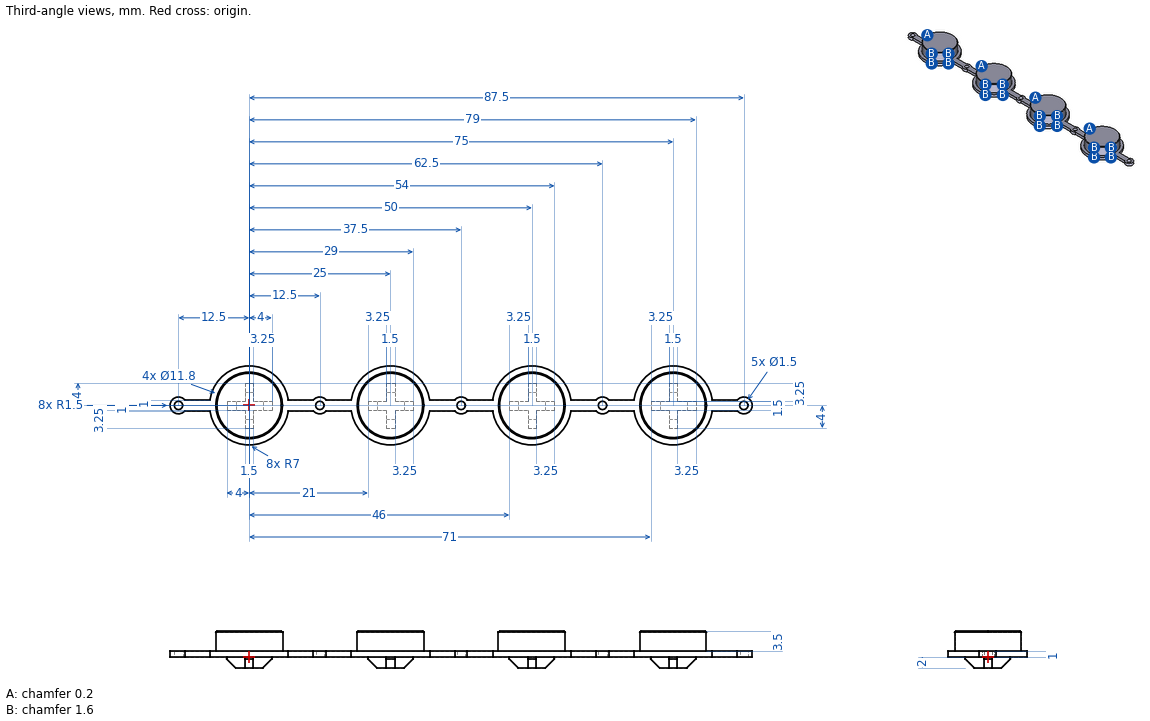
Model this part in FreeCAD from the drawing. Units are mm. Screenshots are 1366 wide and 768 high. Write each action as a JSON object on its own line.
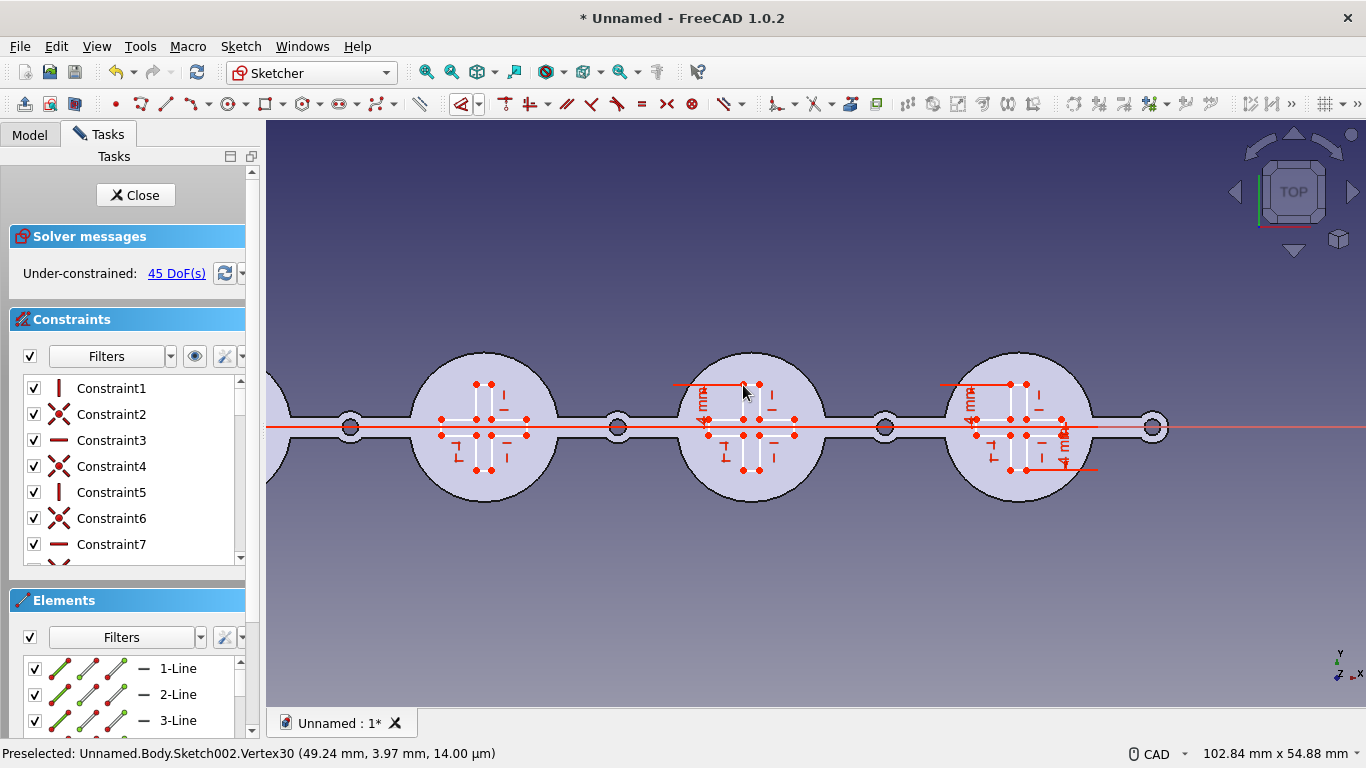
{"action": "left_click", "coordinate": [760, 471]}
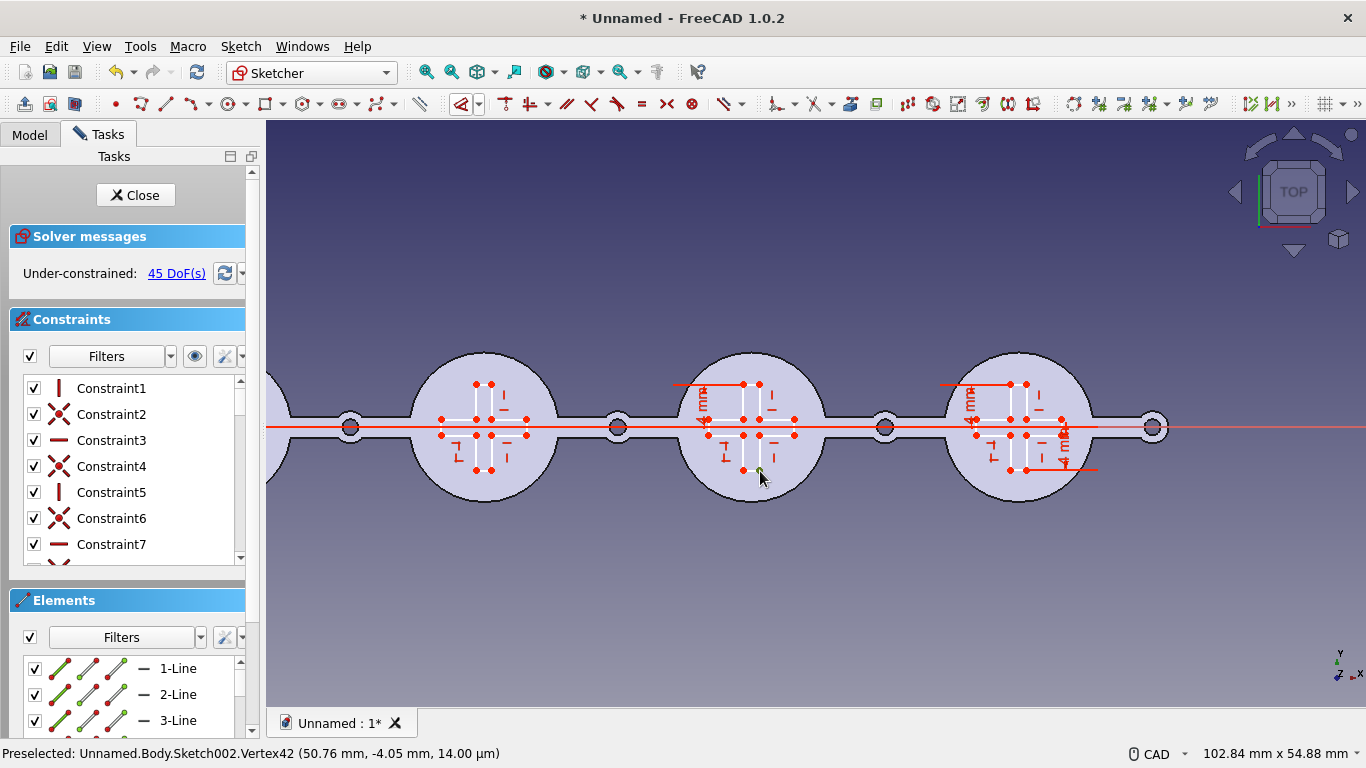
{"action": "left_click", "coordinate": [478, 104]}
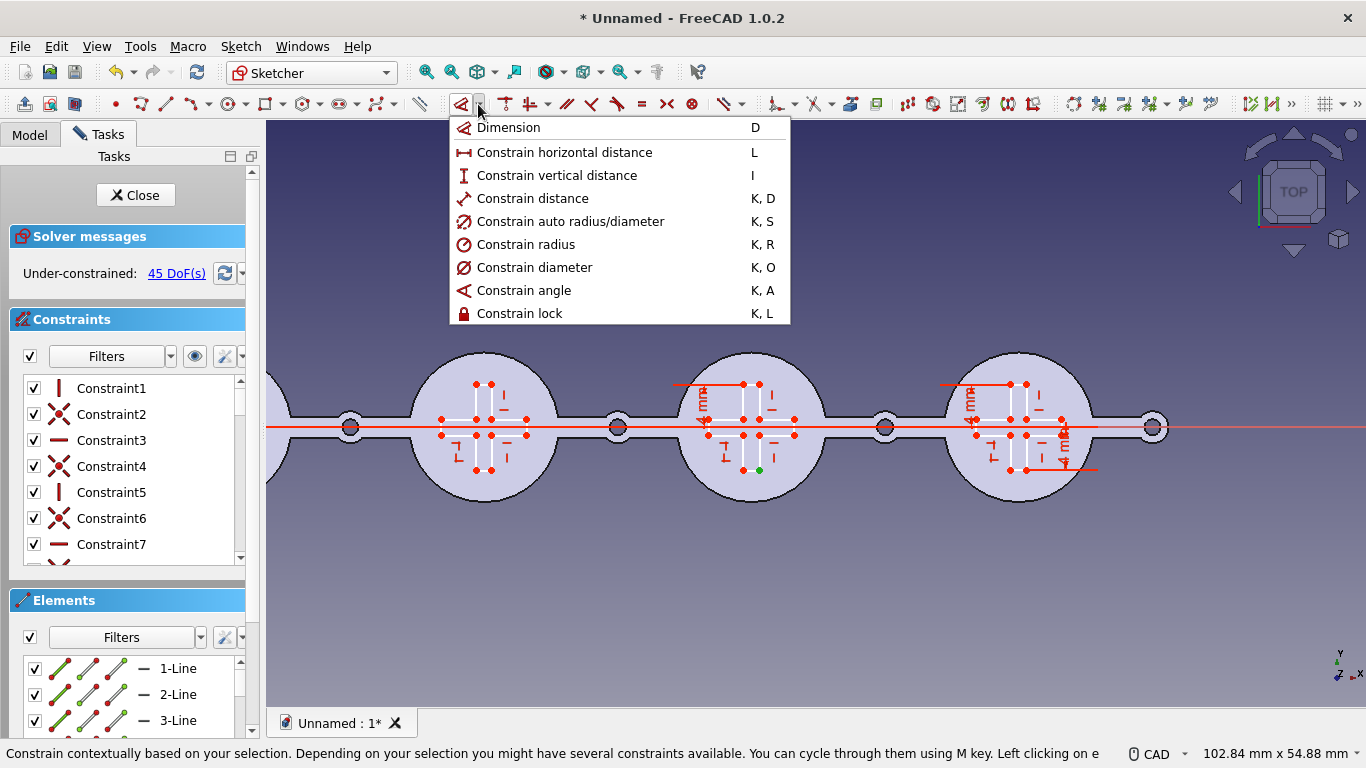
{"action": "left_click", "coordinate": [620, 176]}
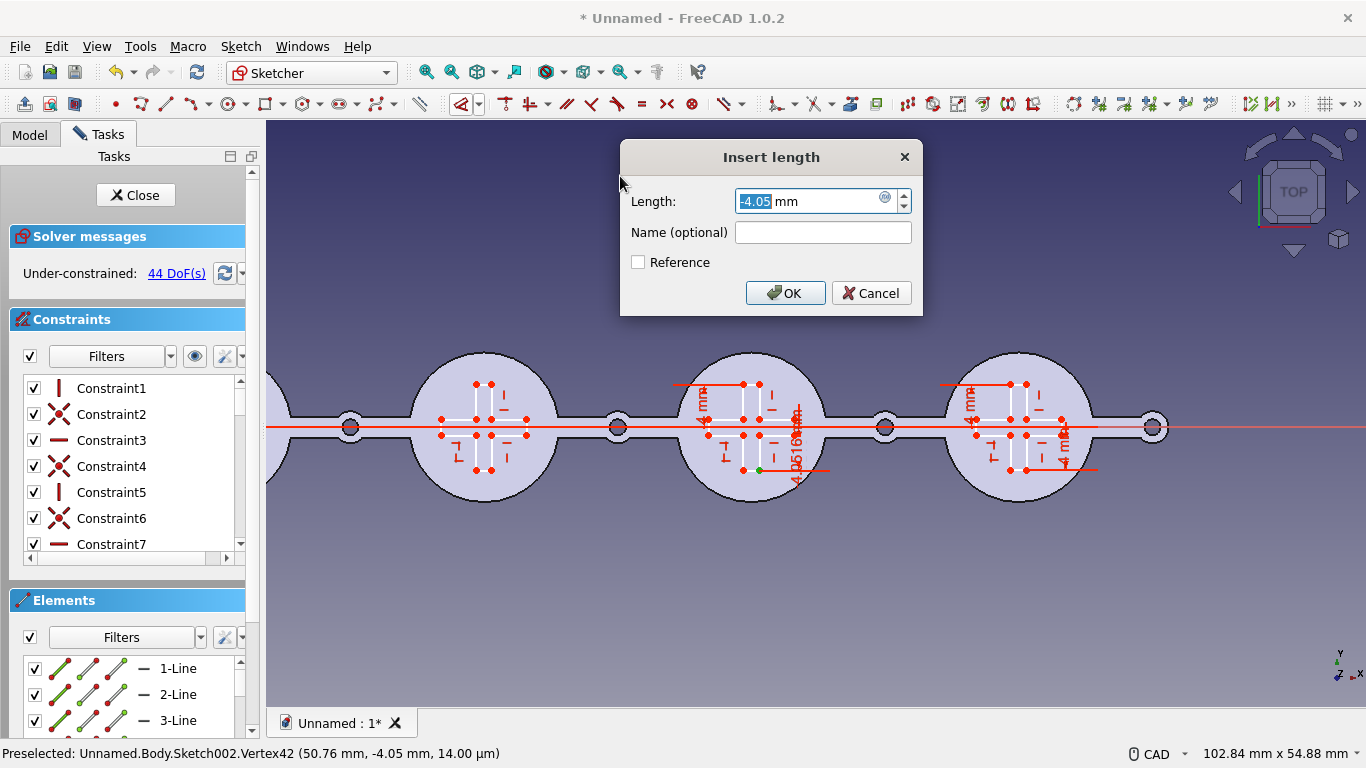
{"action": "type", "text": "-4"}
{"action": "key", "text": "Return"}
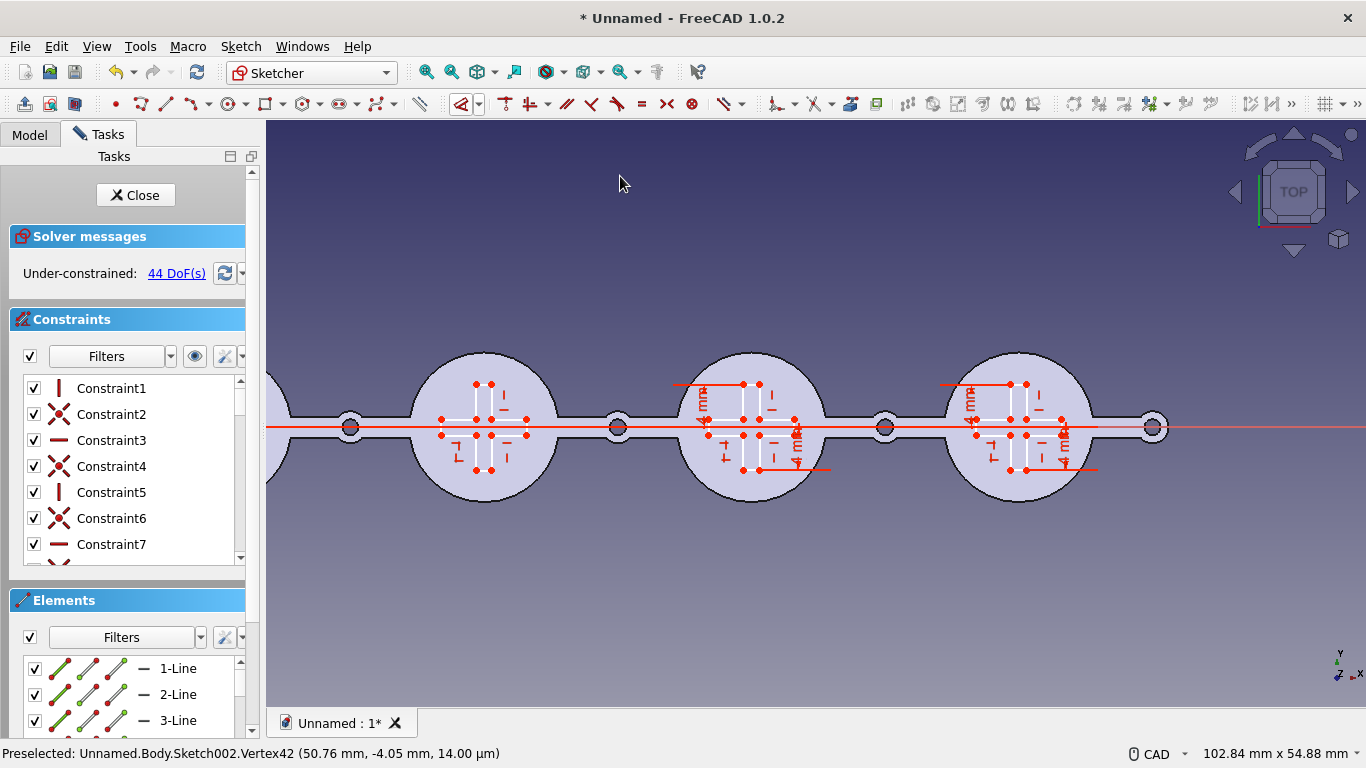
{"action": "left_click", "coordinate": [476, 385]}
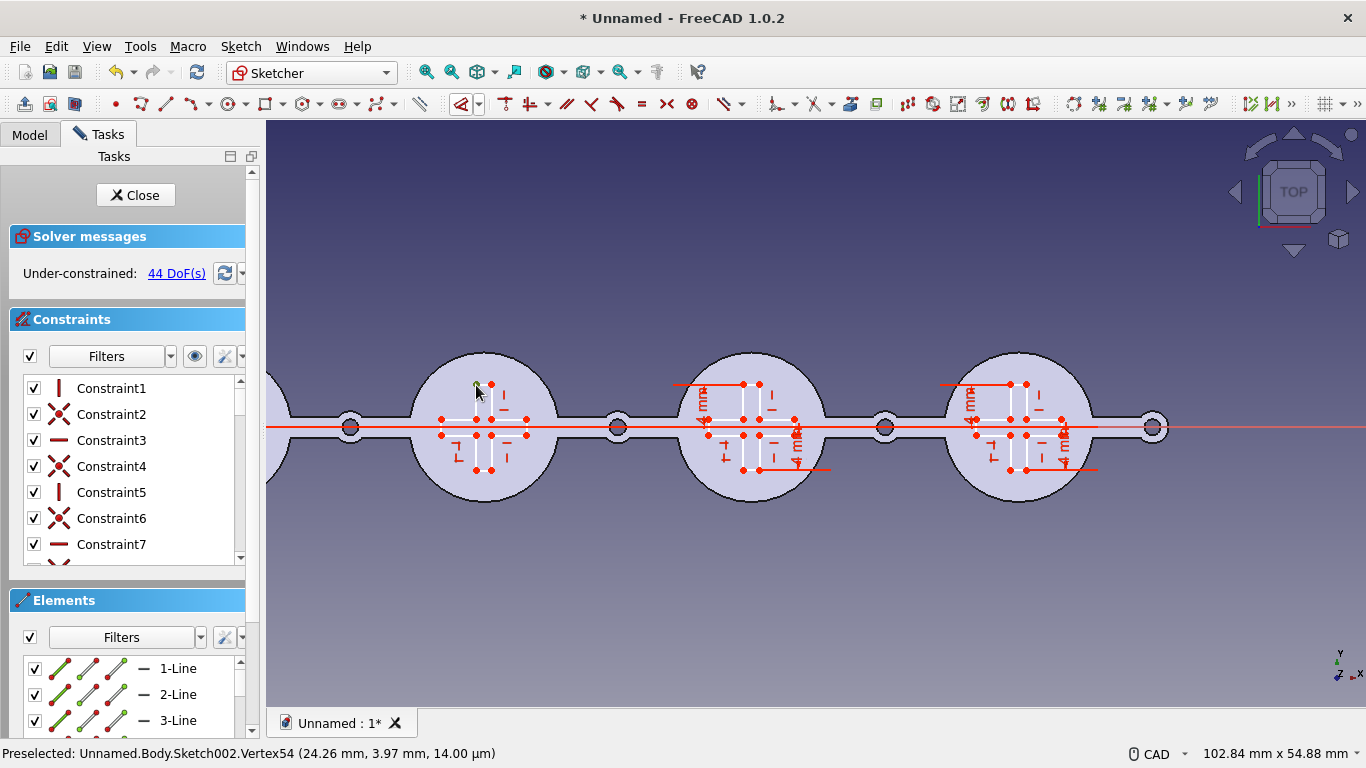
{"action": "key", "text": "i"}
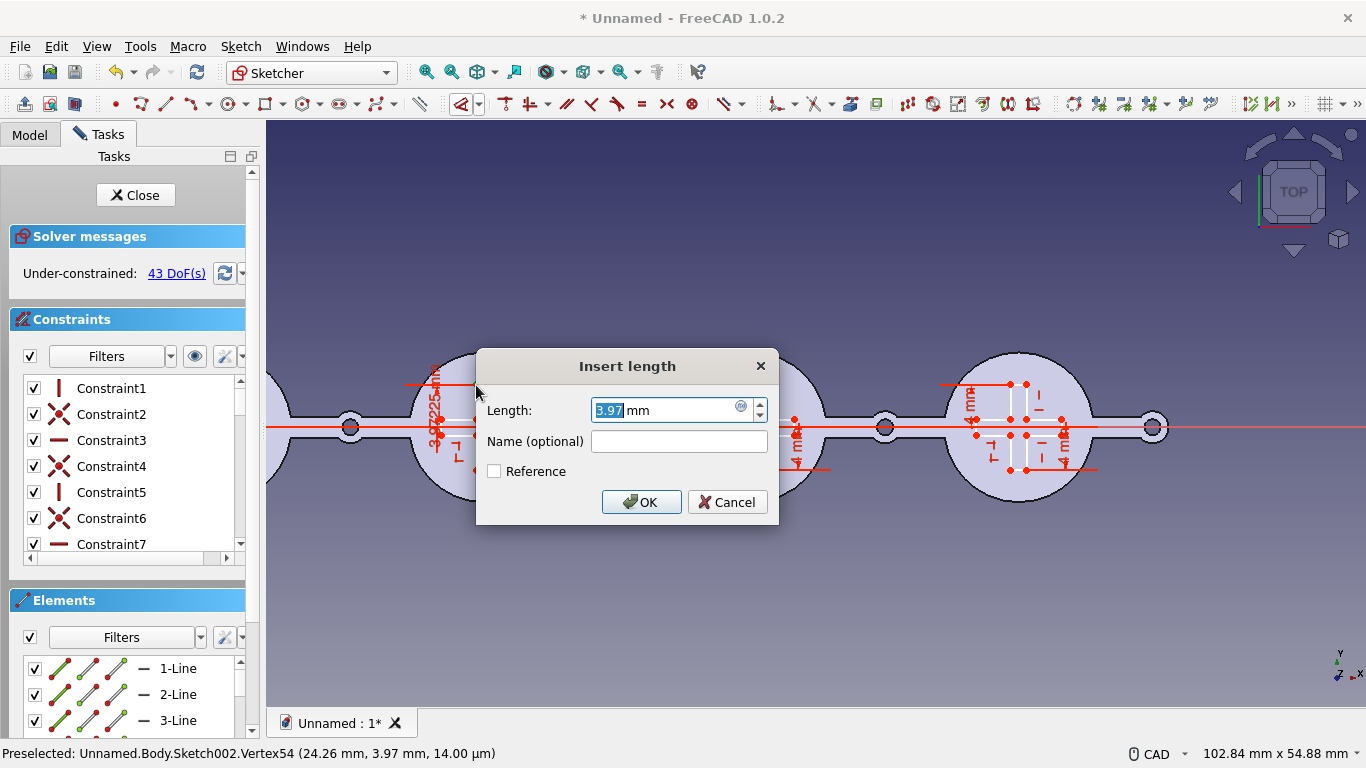
{"action": "type", "text": "4"}
{"action": "key", "text": "Return"}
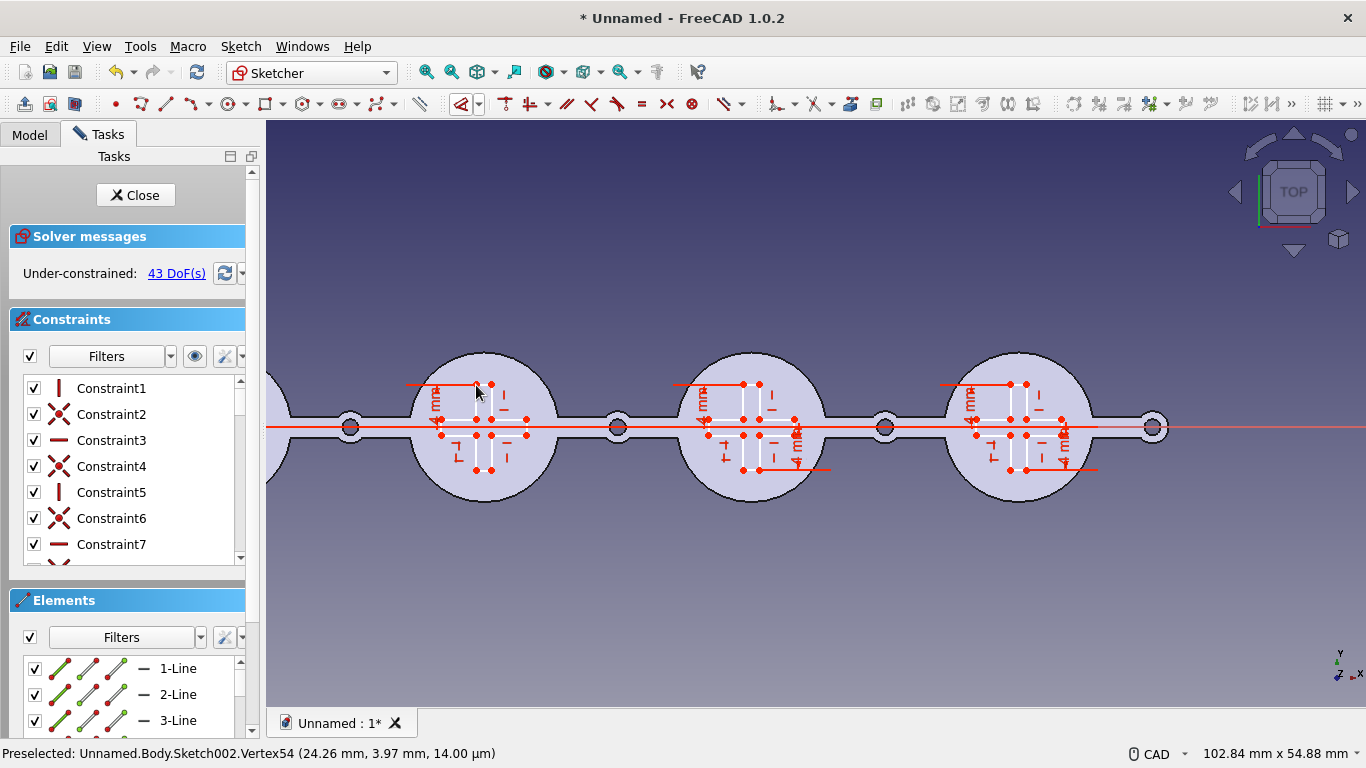
{"action": "left_click", "coordinate": [492, 471]}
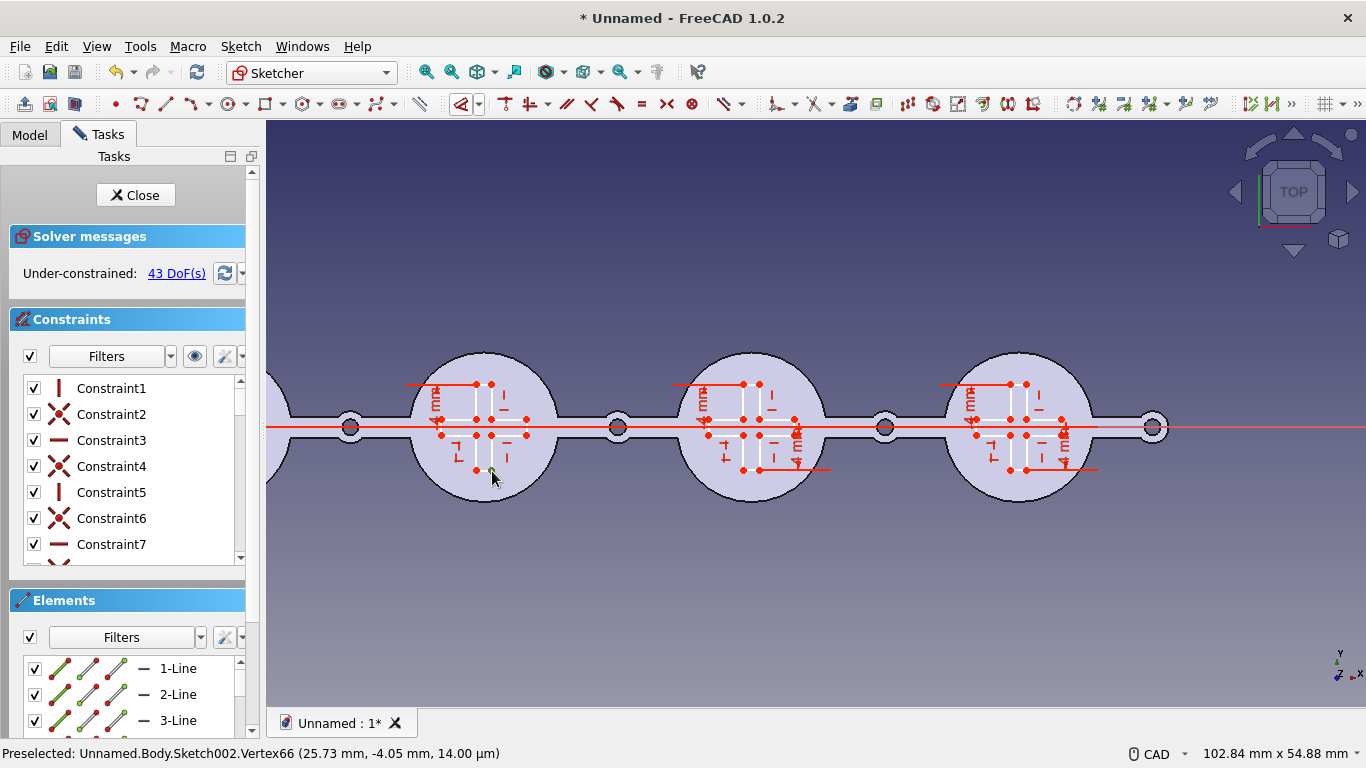
{"action": "left_click", "coordinate": [478, 104]}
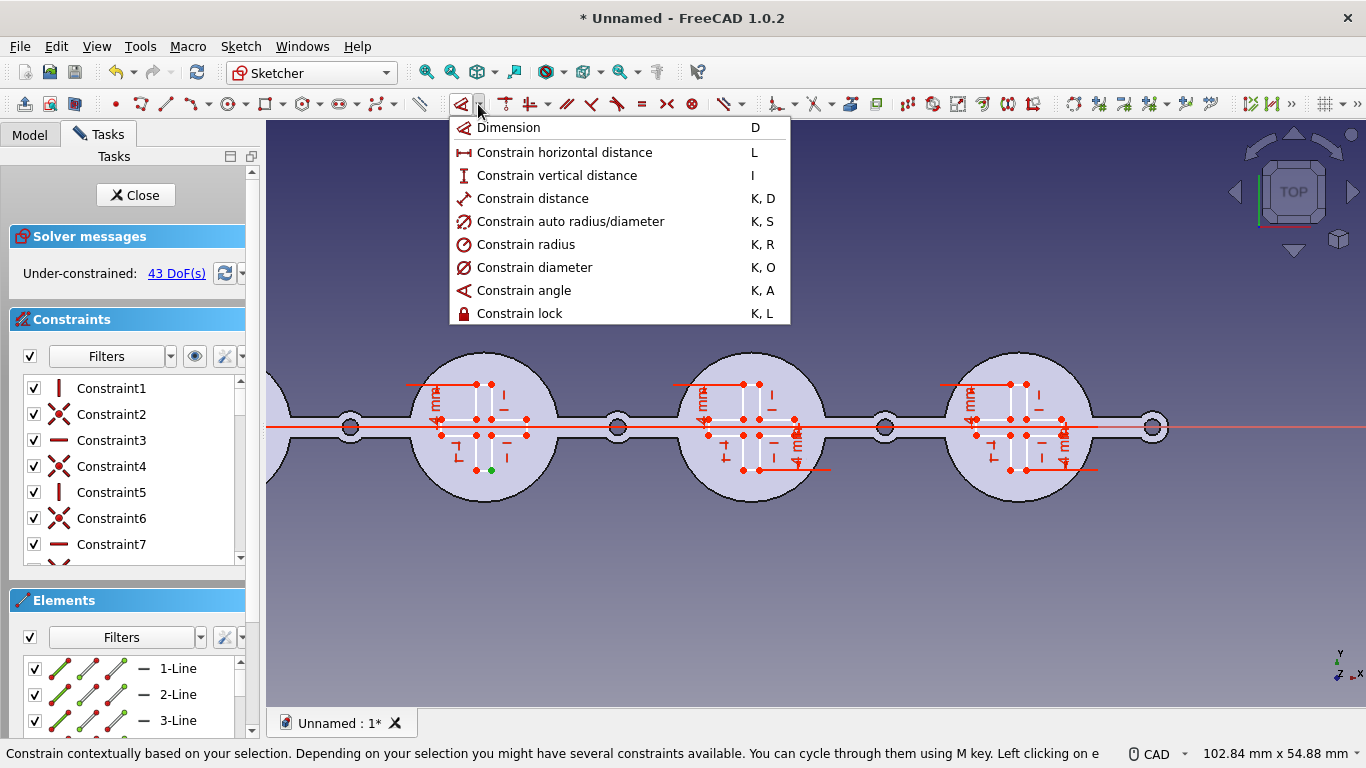
{"action": "left_click", "coordinate": [620, 176]}